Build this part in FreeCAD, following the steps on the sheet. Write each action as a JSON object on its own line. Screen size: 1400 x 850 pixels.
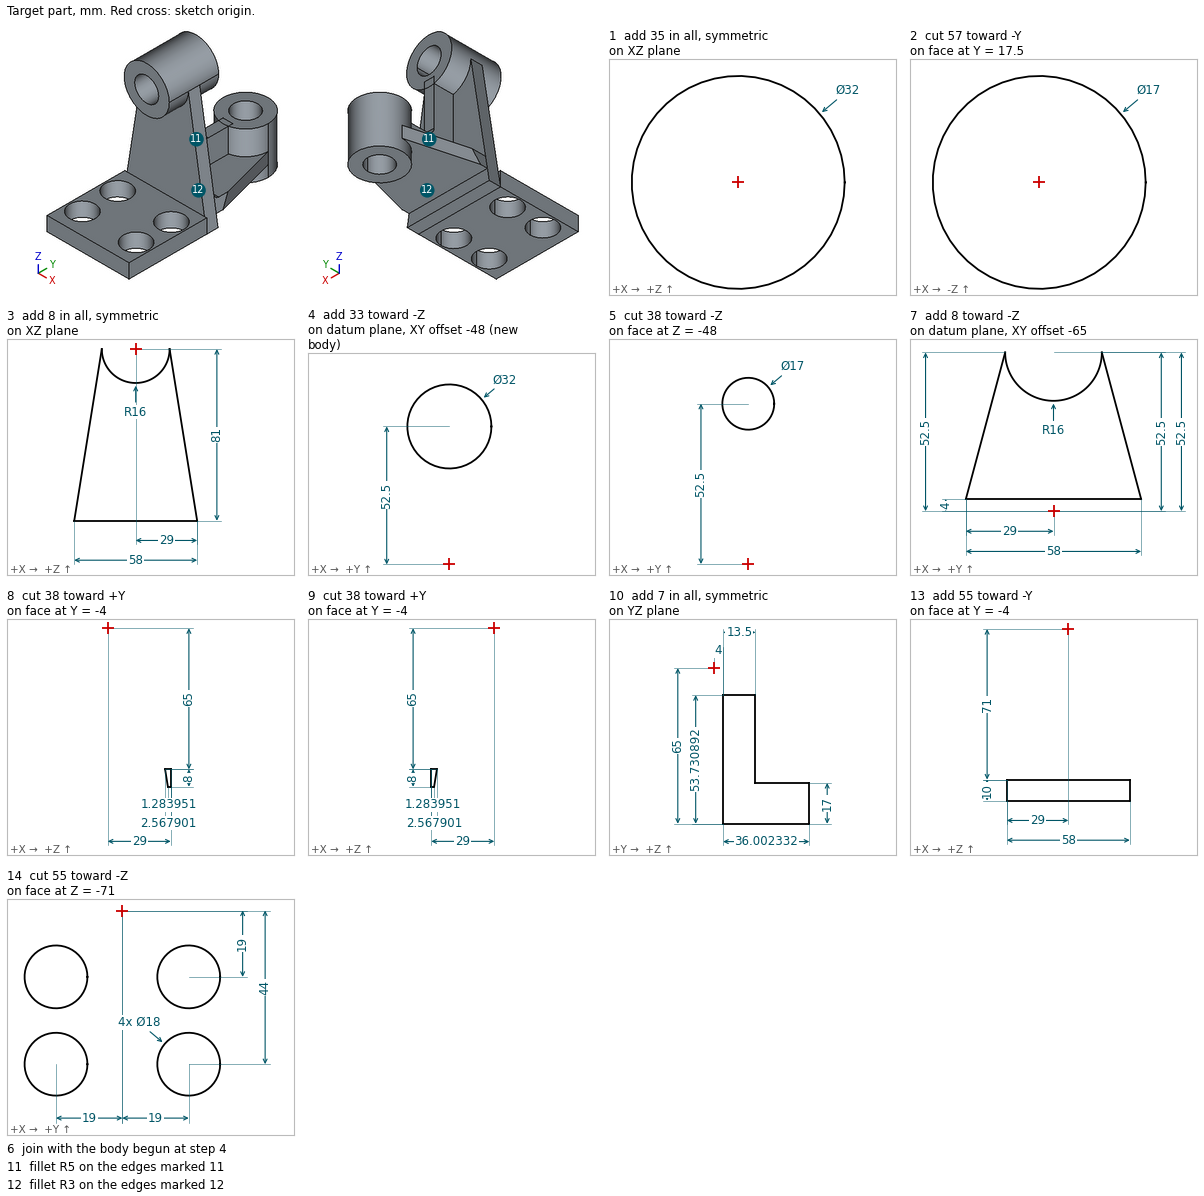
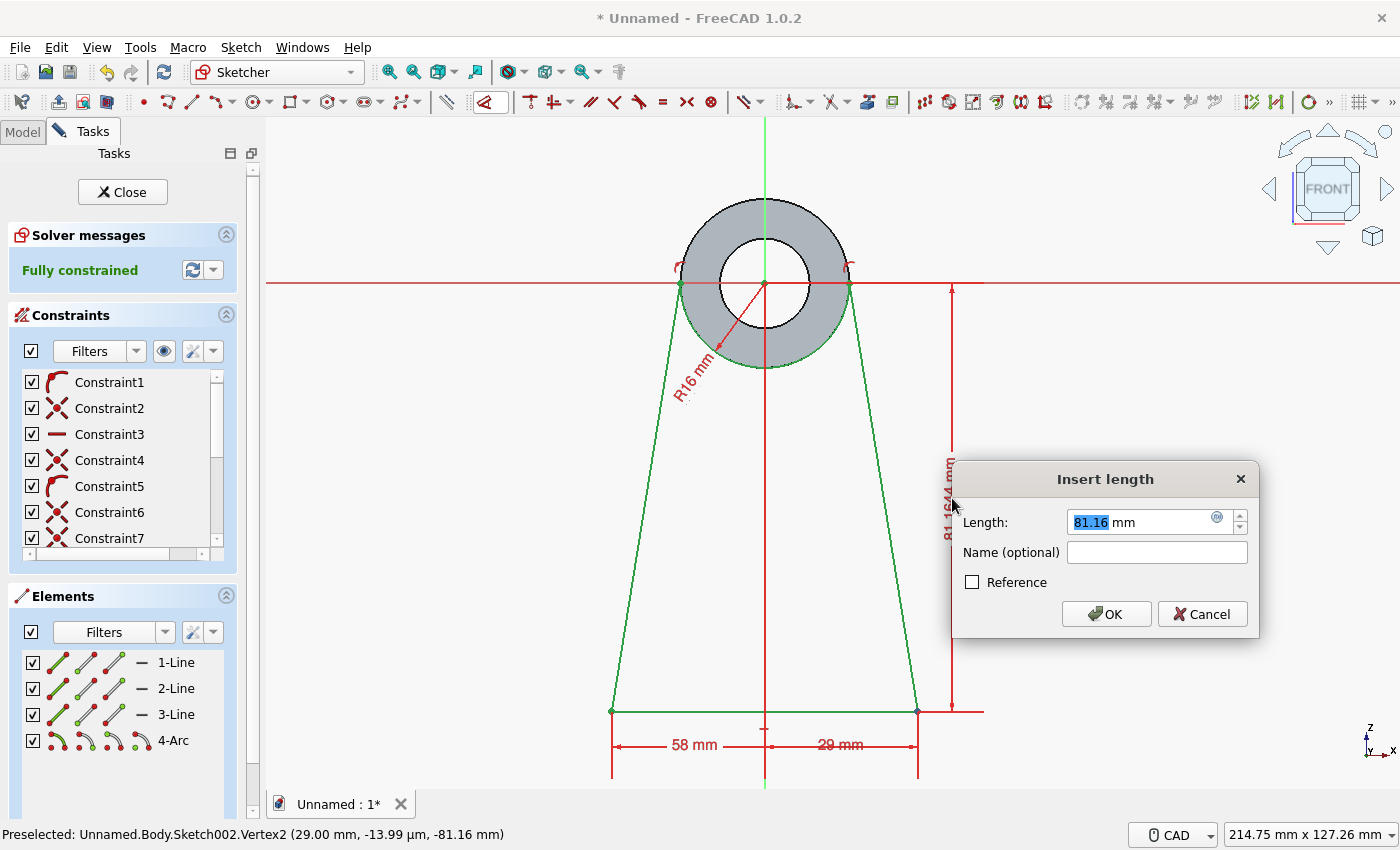
{"action": "type", "text": "81"}
{"action": "key", "text": "Return"}
{"action": "key", "text": "Escape"}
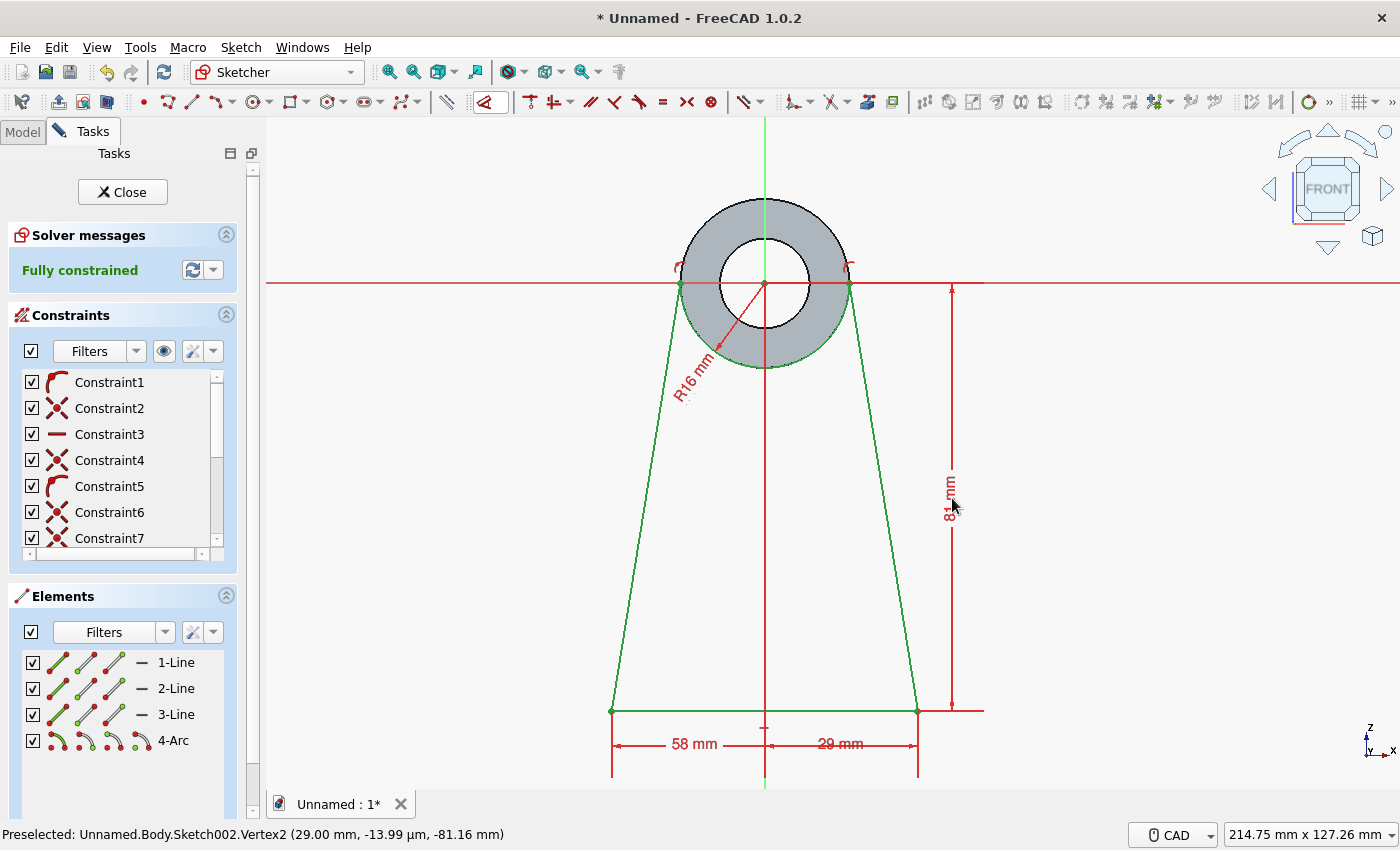
{"action": "left_click", "coordinate": [123, 192]}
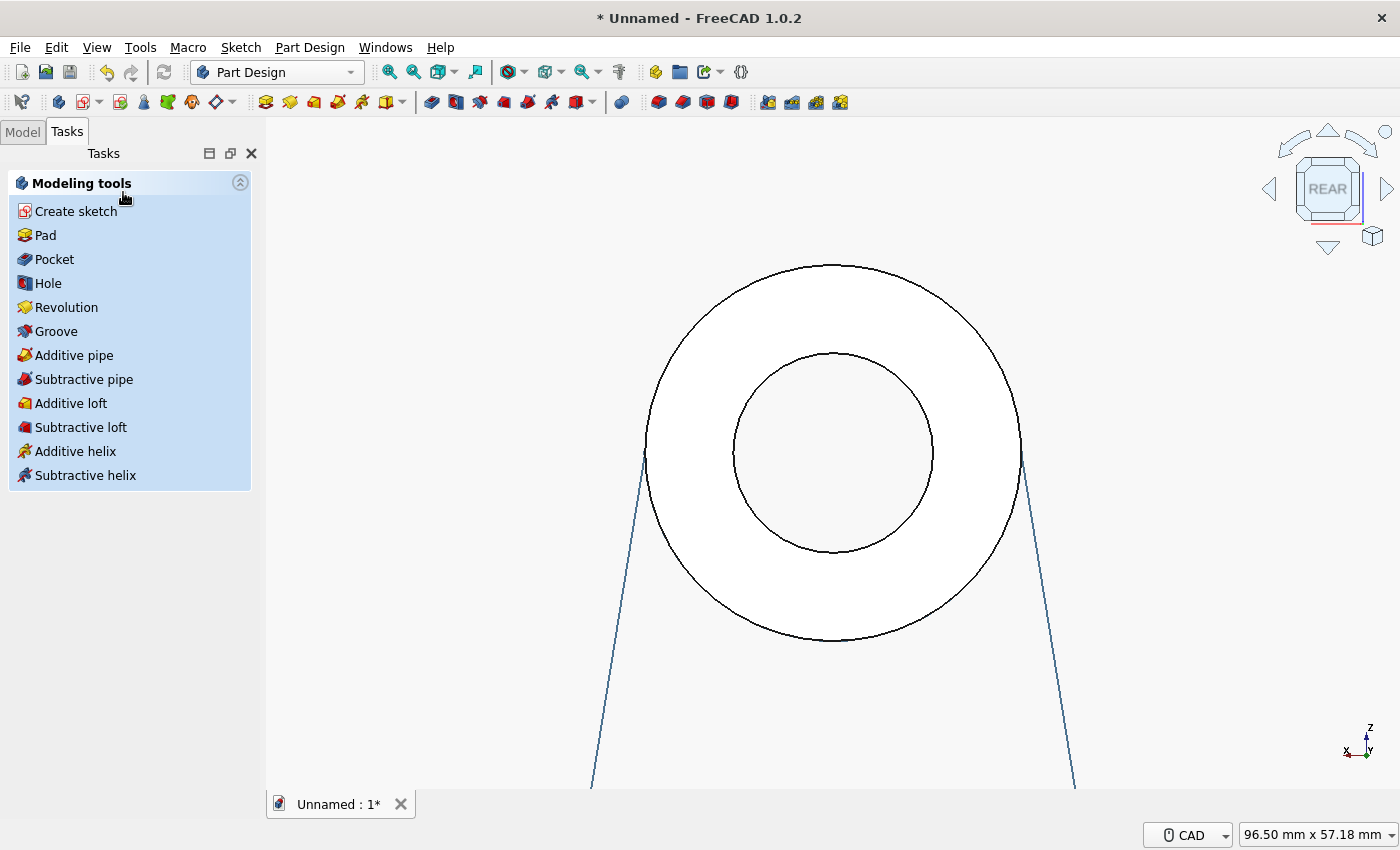
{"action": "left_click", "coordinate": [266, 102]}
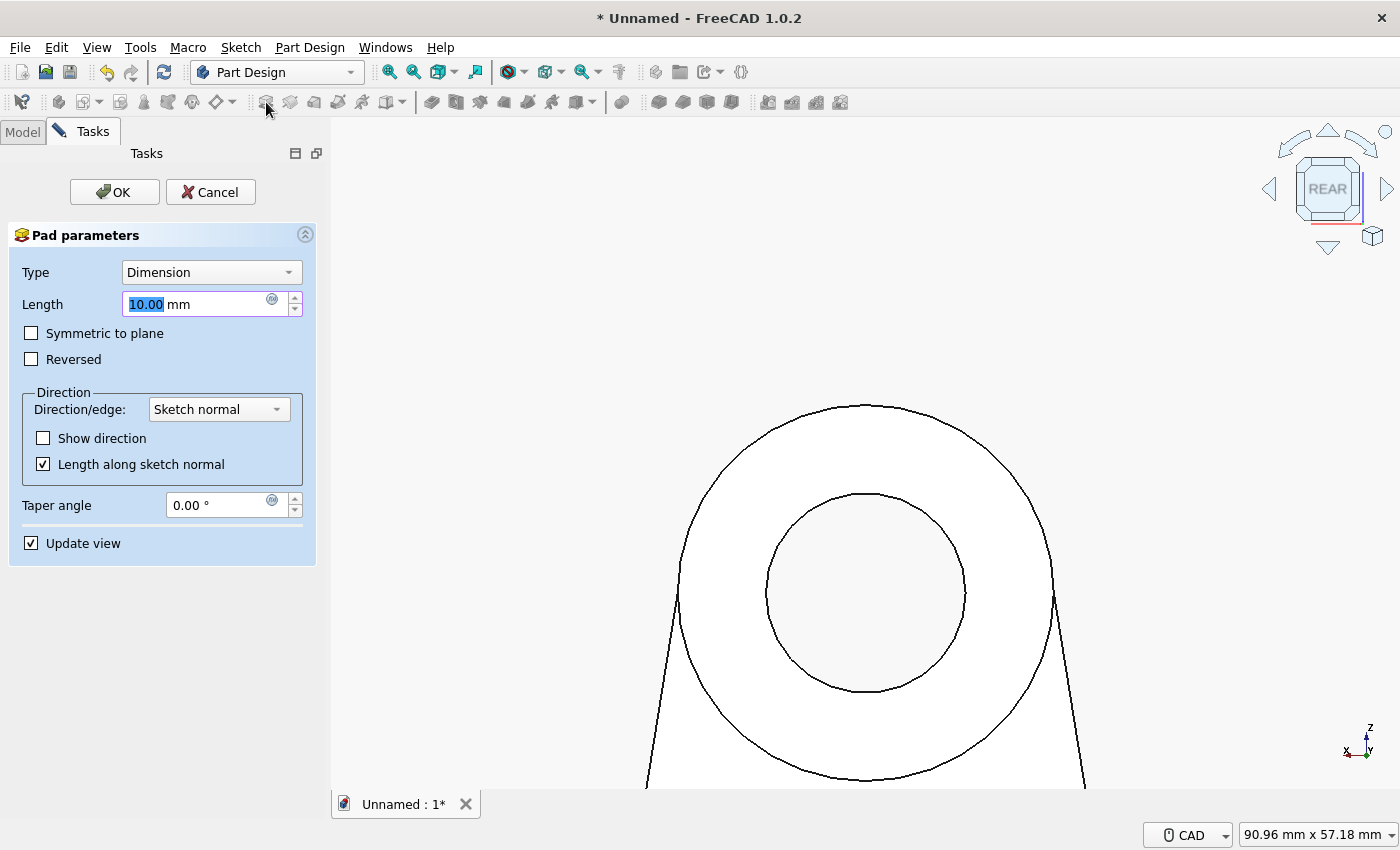
{"action": "type", "text": "8"}
{"action": "key", "text": "Tab"}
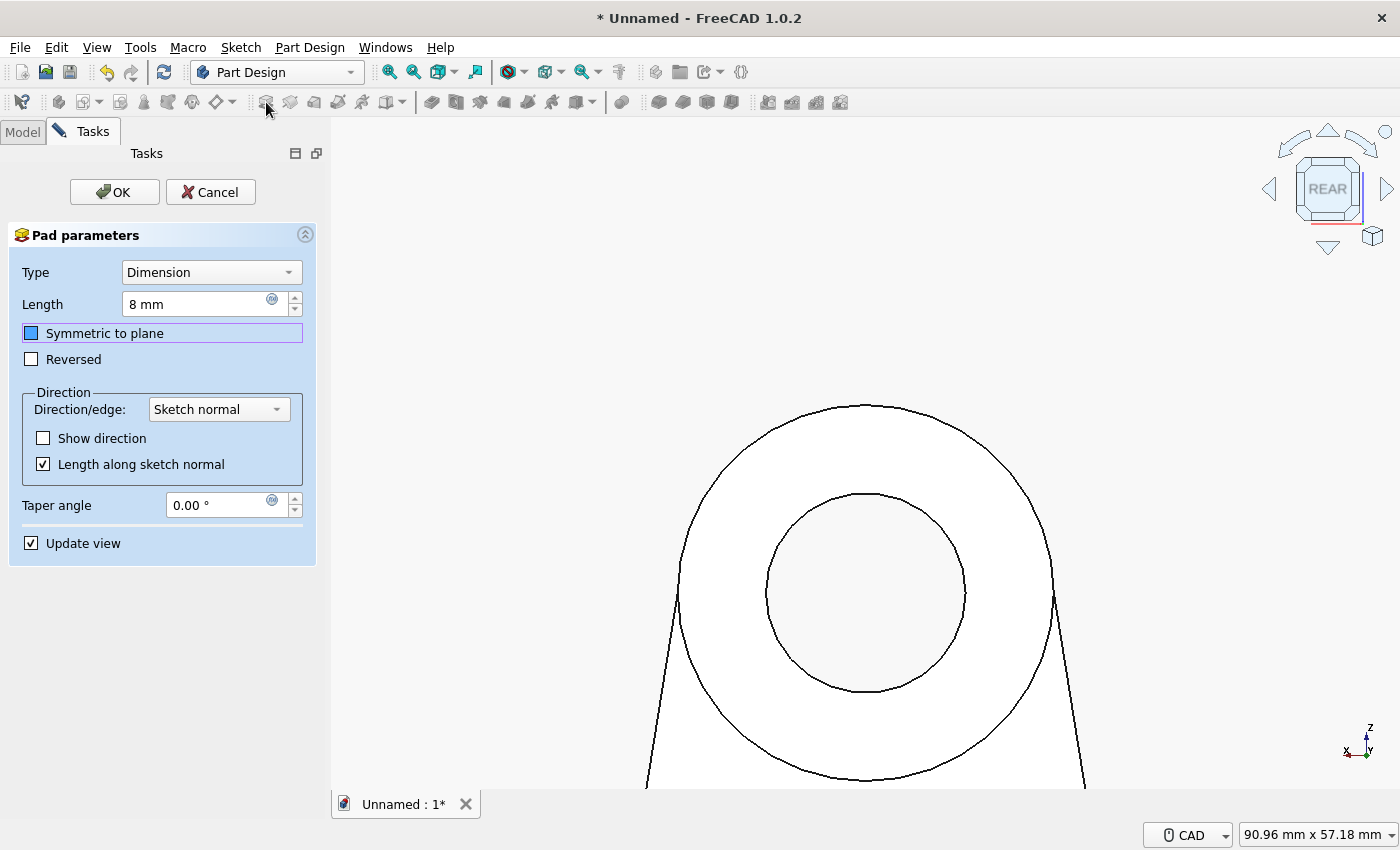
{"action": "left_click", "coordinate": [30, 333]}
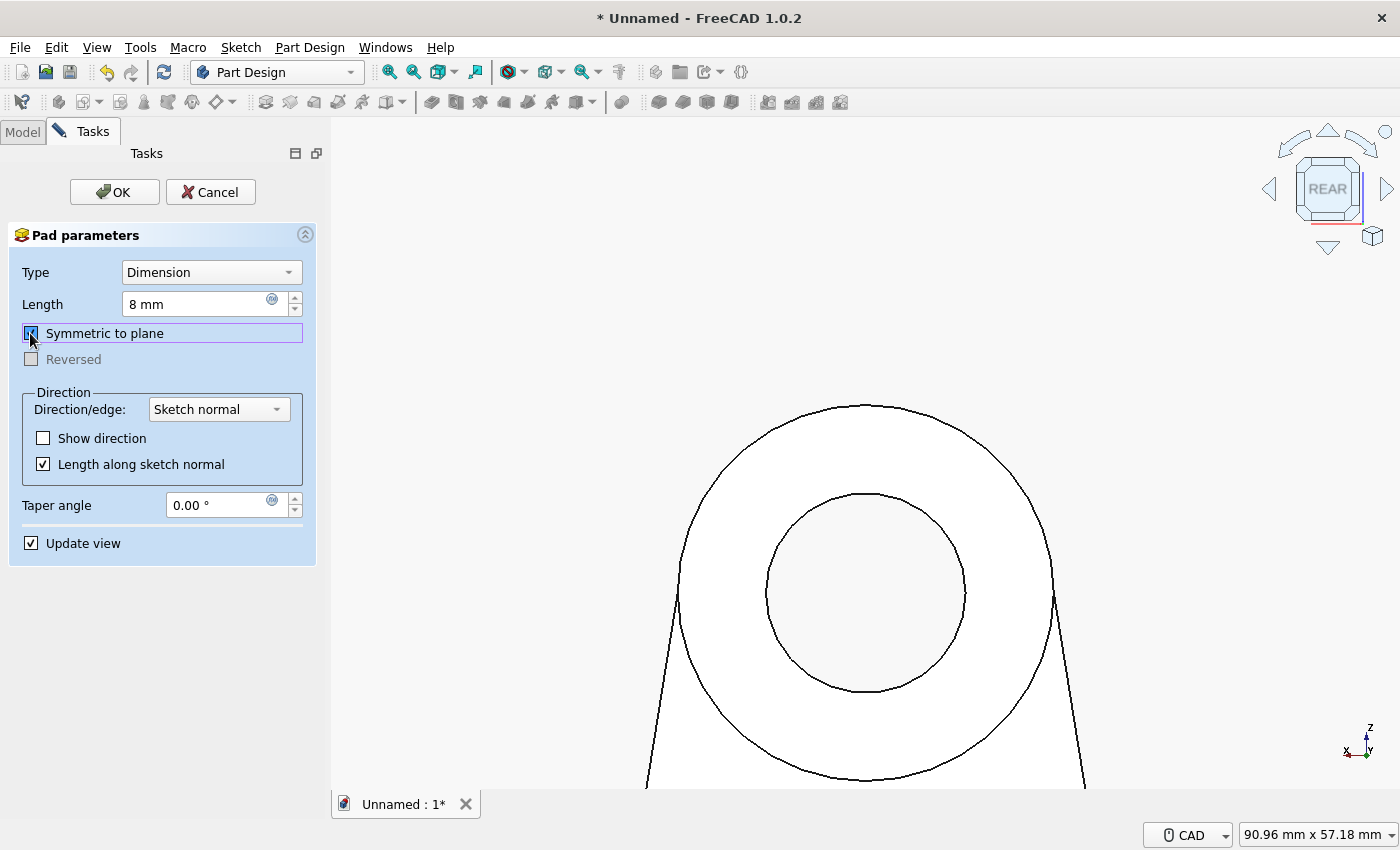
{"action": "left_click", "coordinate": [115, 192]}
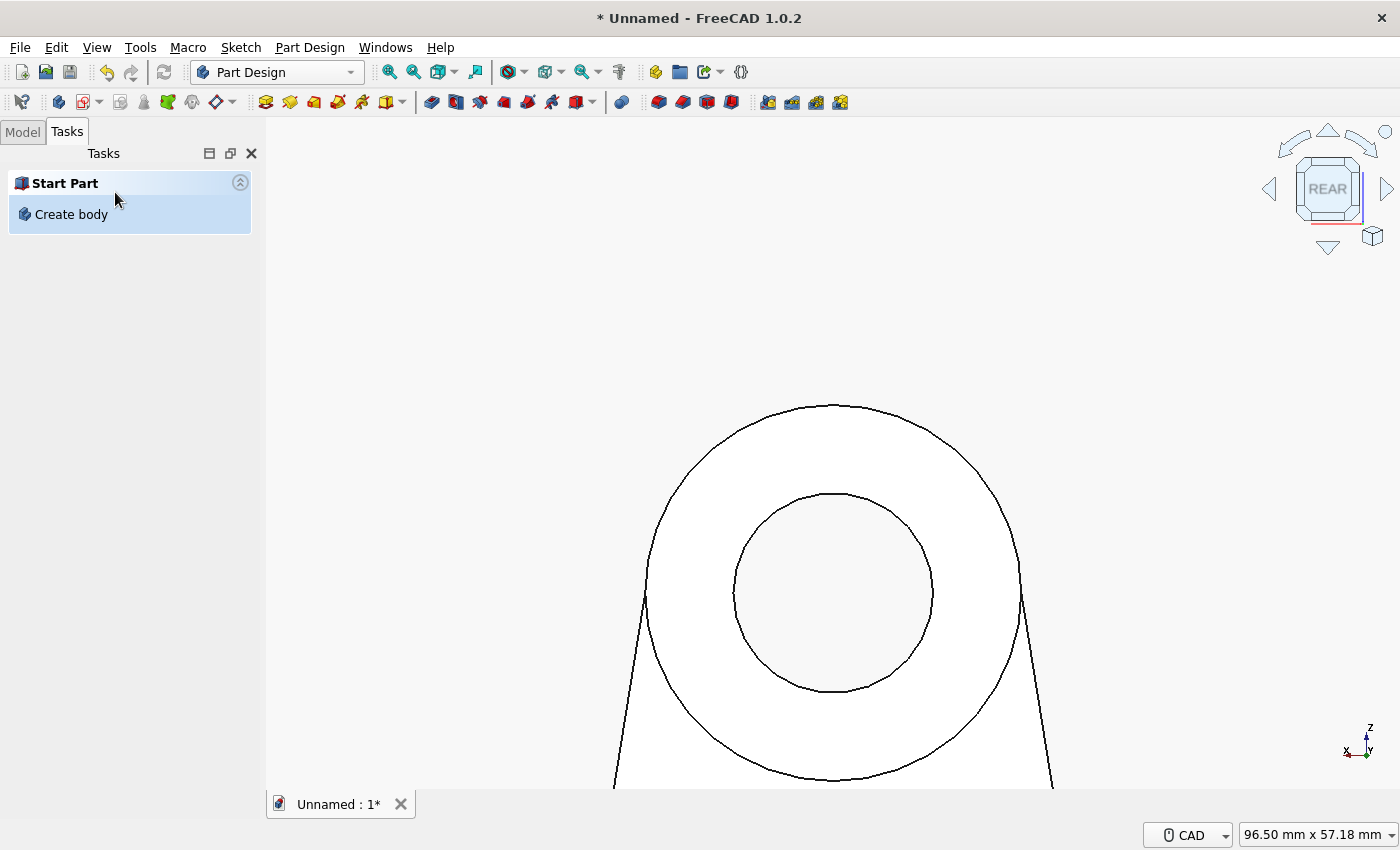
{"action": "key", "text": "v f"}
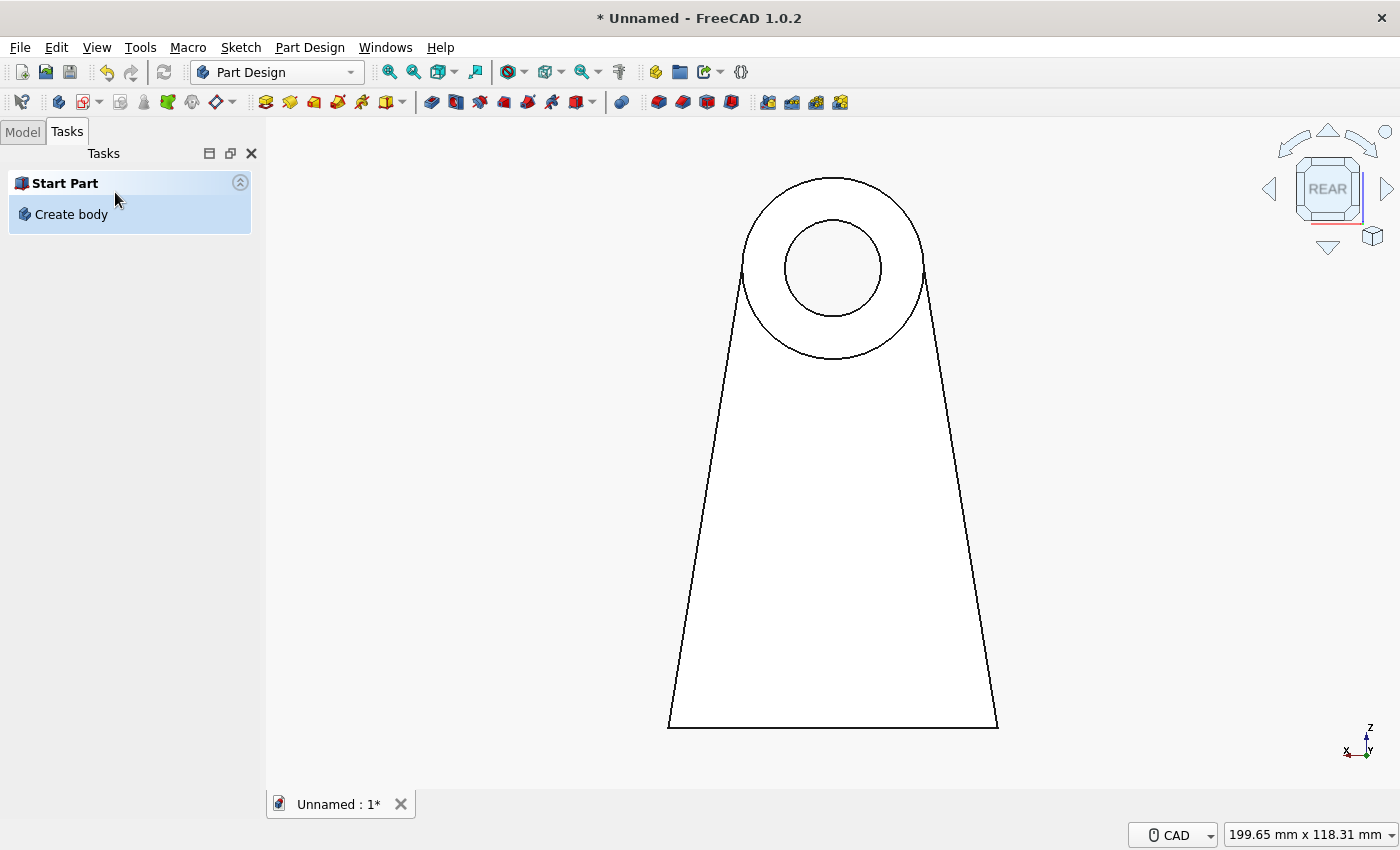
{"action": "left_click", "coordinate": [60, 102]}